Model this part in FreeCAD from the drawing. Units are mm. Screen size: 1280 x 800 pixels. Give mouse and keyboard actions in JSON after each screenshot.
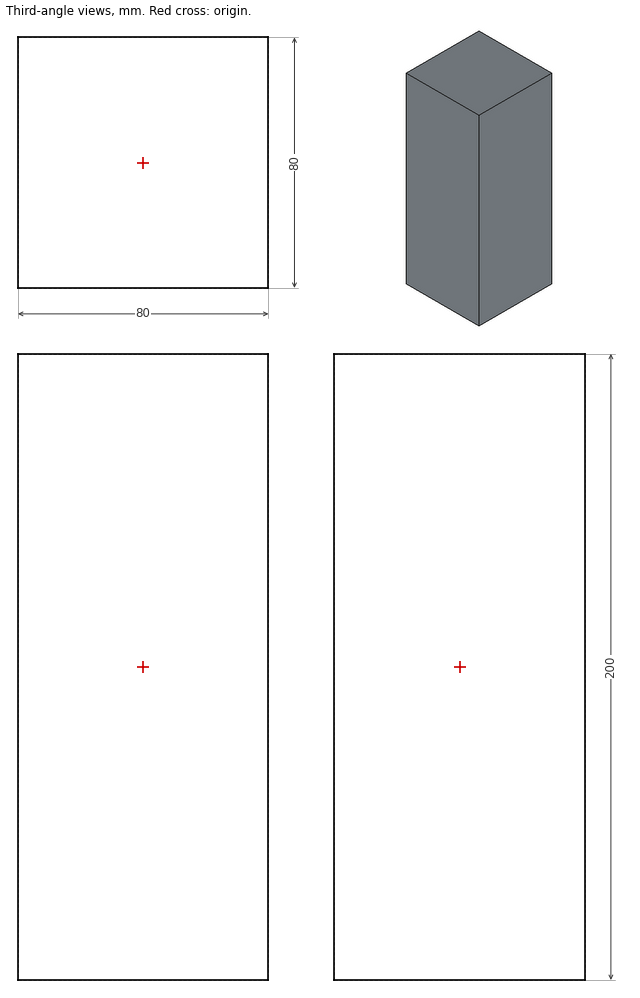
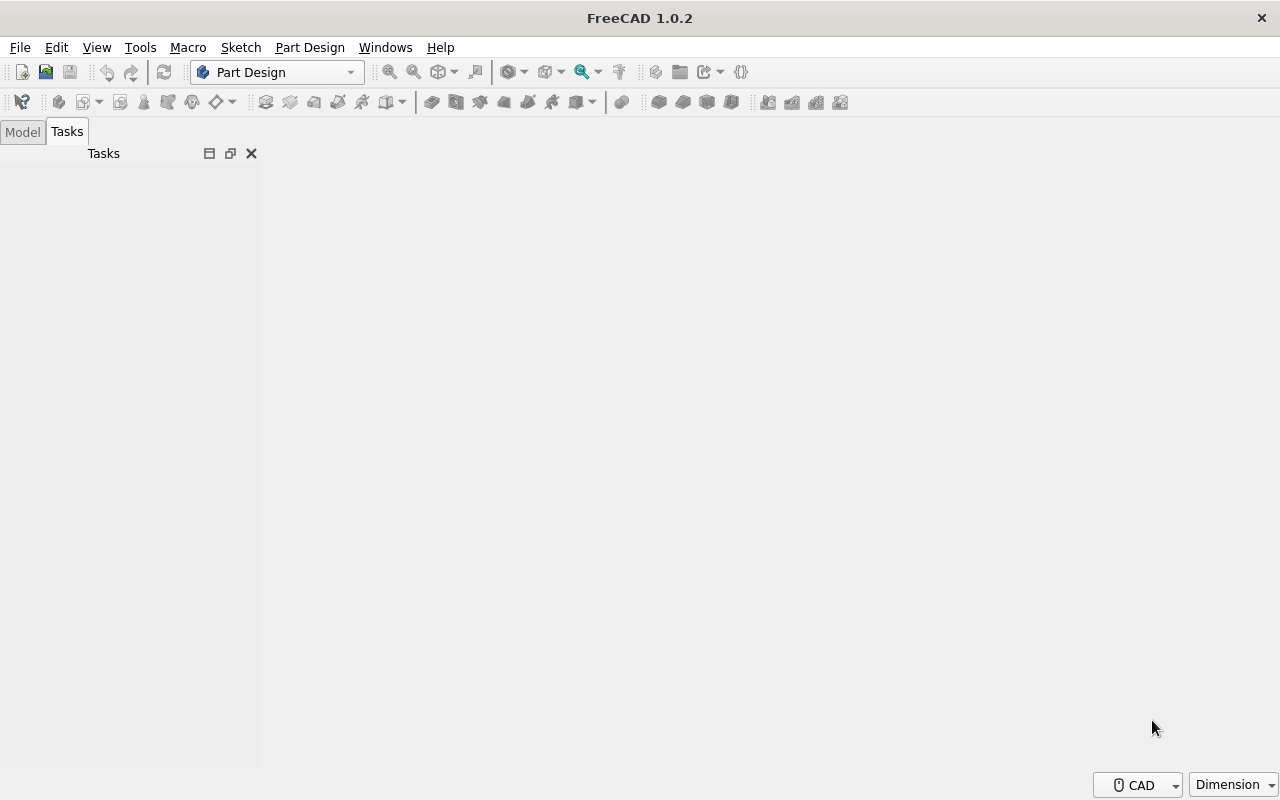
{"action": "left_click", "coordinate": [22, 72]}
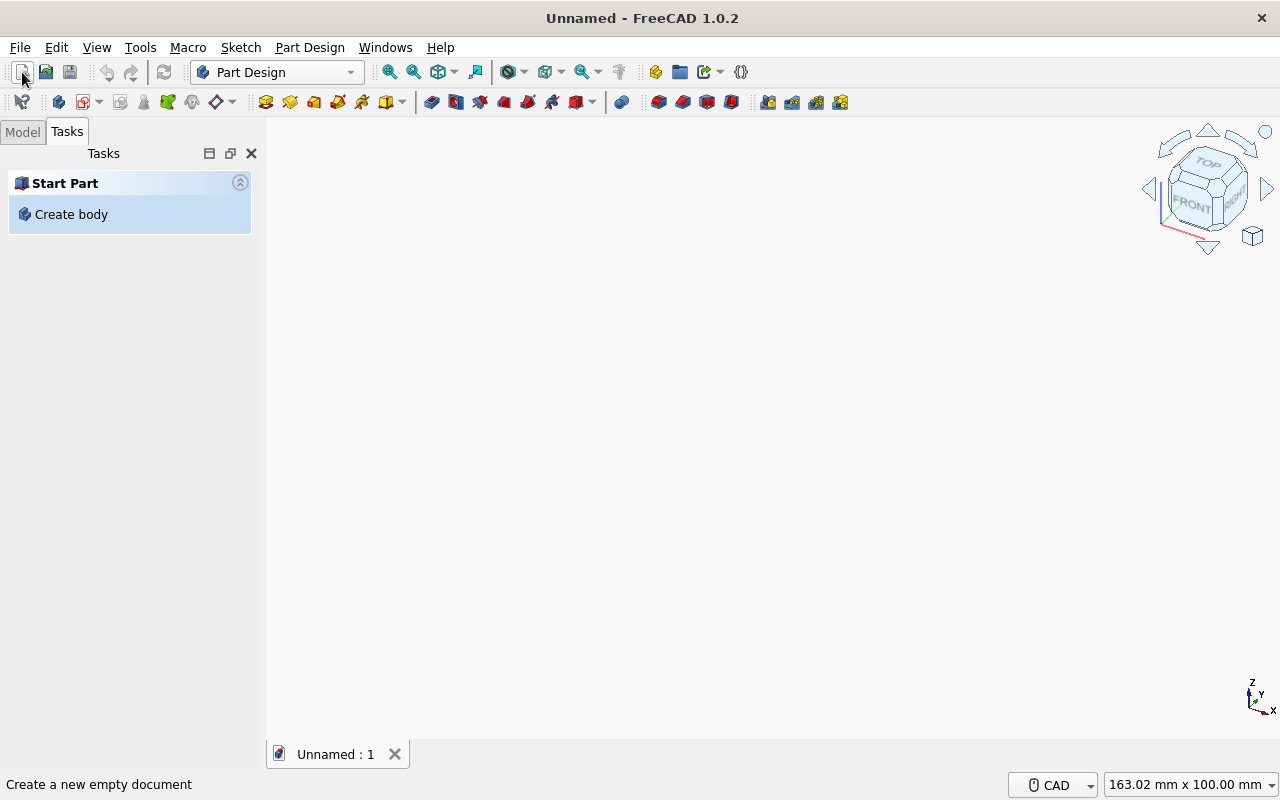
{"action": "left_click", "coordinate": [84, 102]}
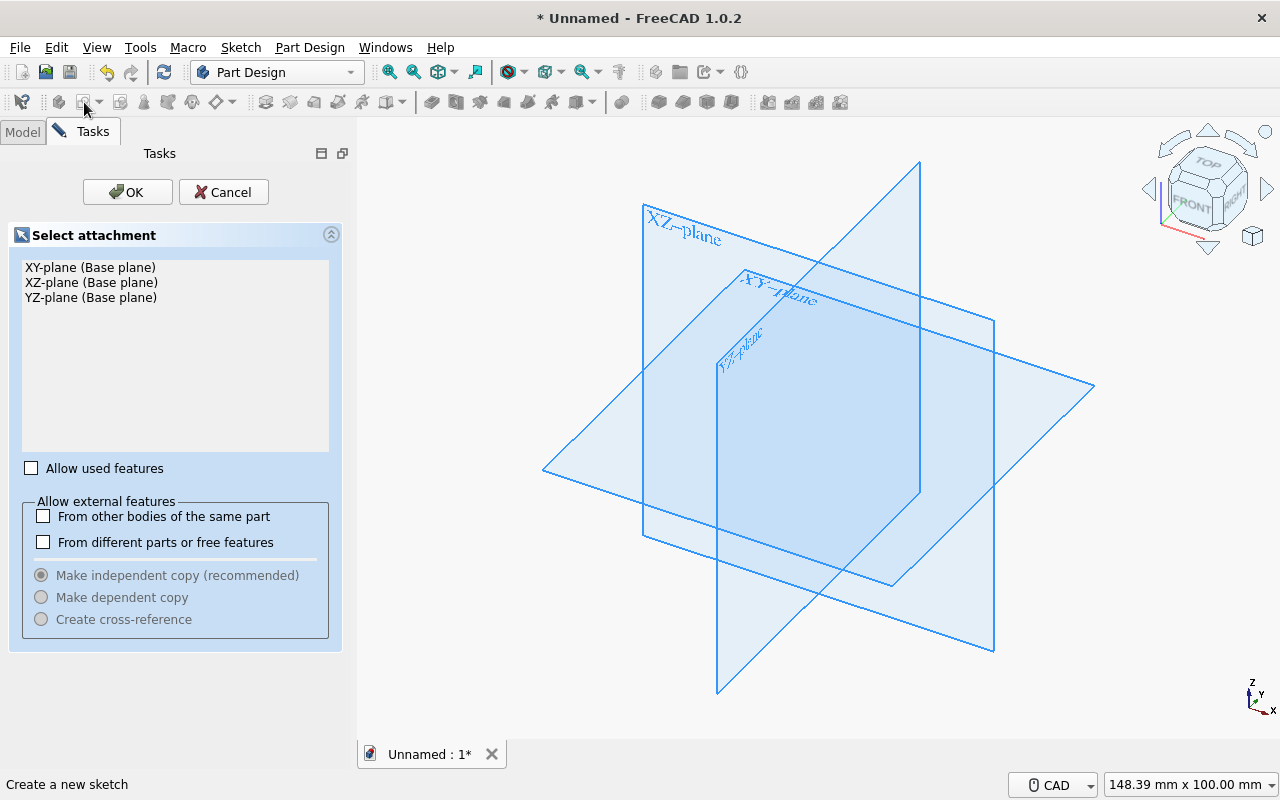
{"action": "left_click", "coordinate": [82, 268]}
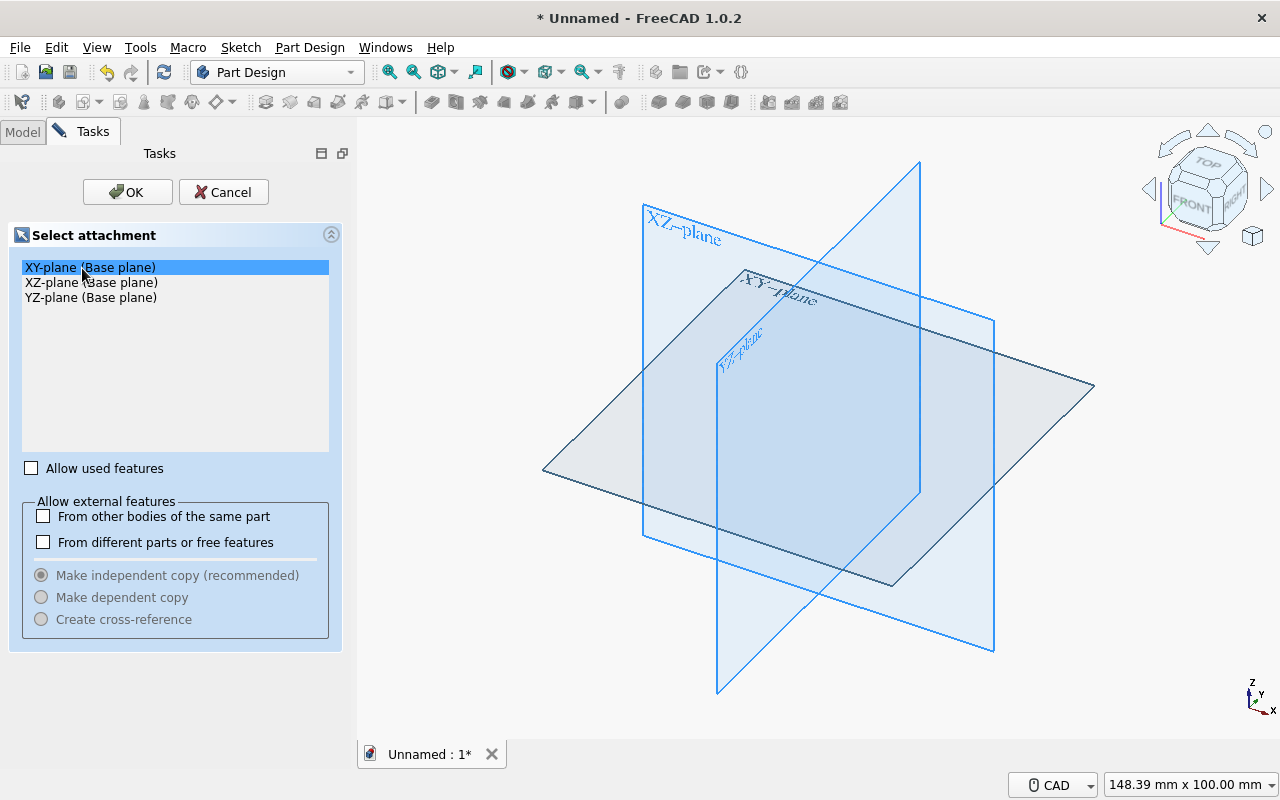
{"action": "left_click", "coordinate": [128, 192]}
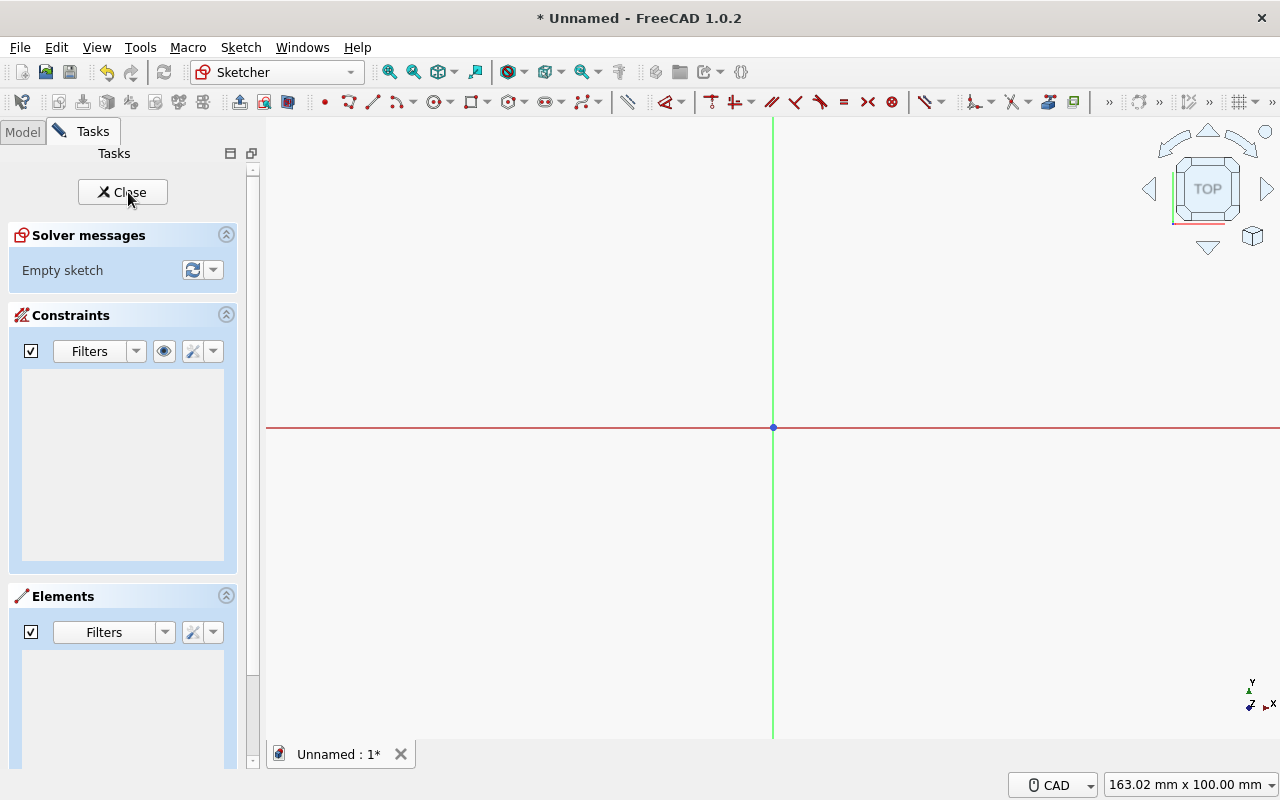
{"action": "key", "text": "g v"}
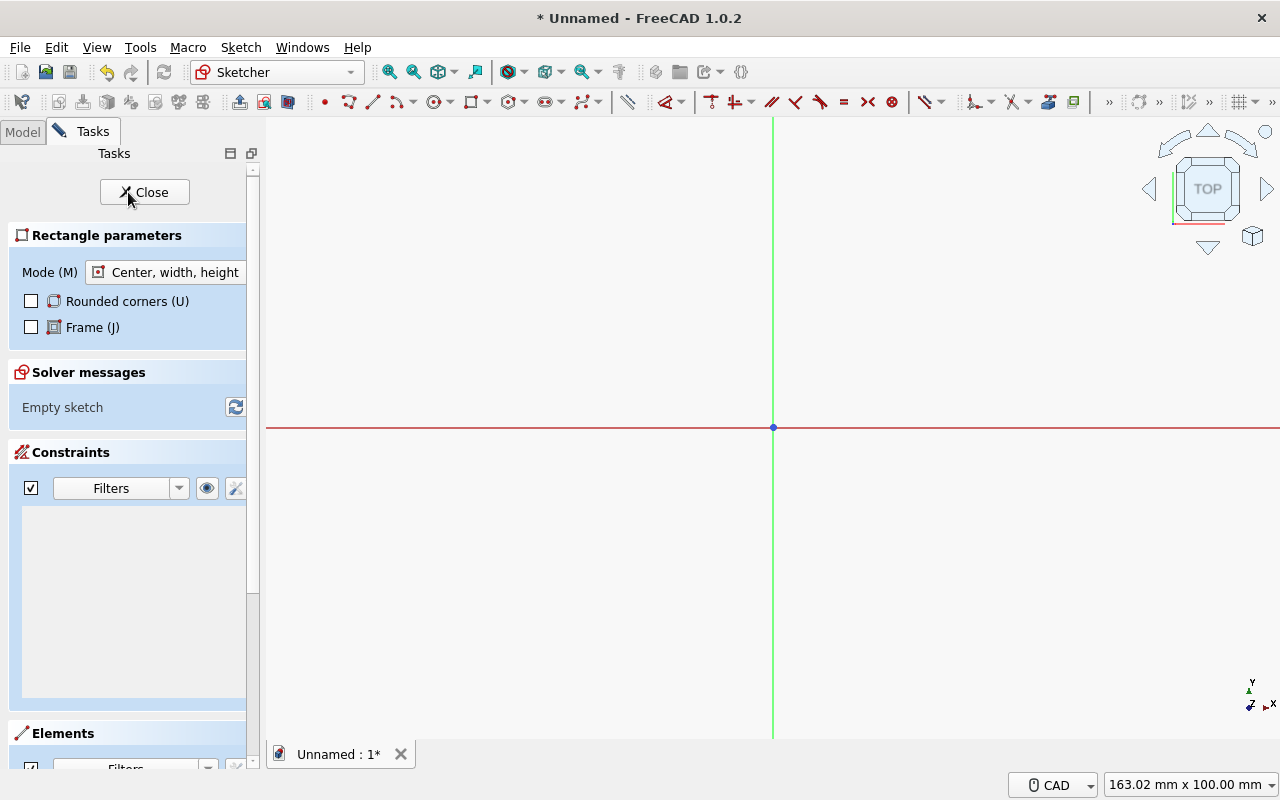
{"action": "left_click", "coordinate": [773, 428]}
{"action": "mouse_move", "coordinate": [1022, 179]}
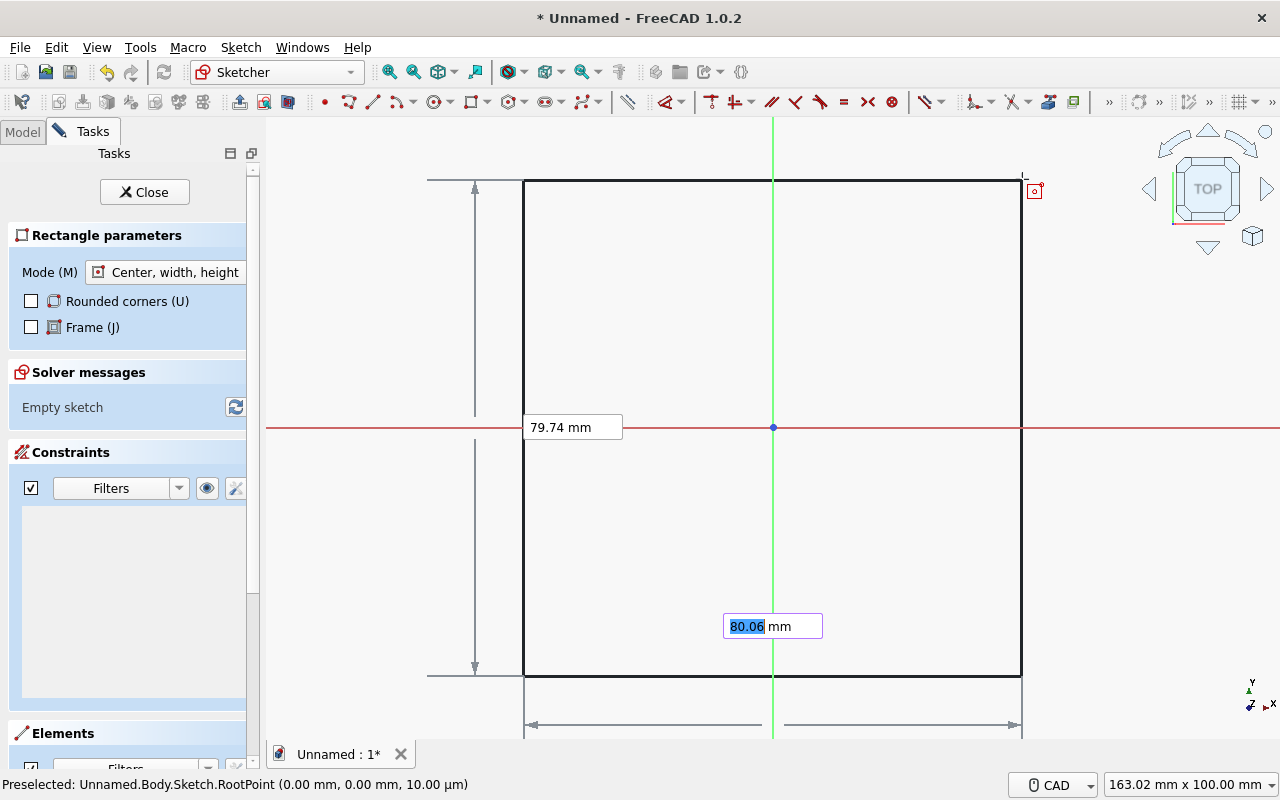
{"action": "type", "text": "80"}
{"action": "key", "text": "Tab"}
{"action": "type", "text": "80"}
{"action": "key", "text": "Return"}
{"action": "key", "text": "Escape"}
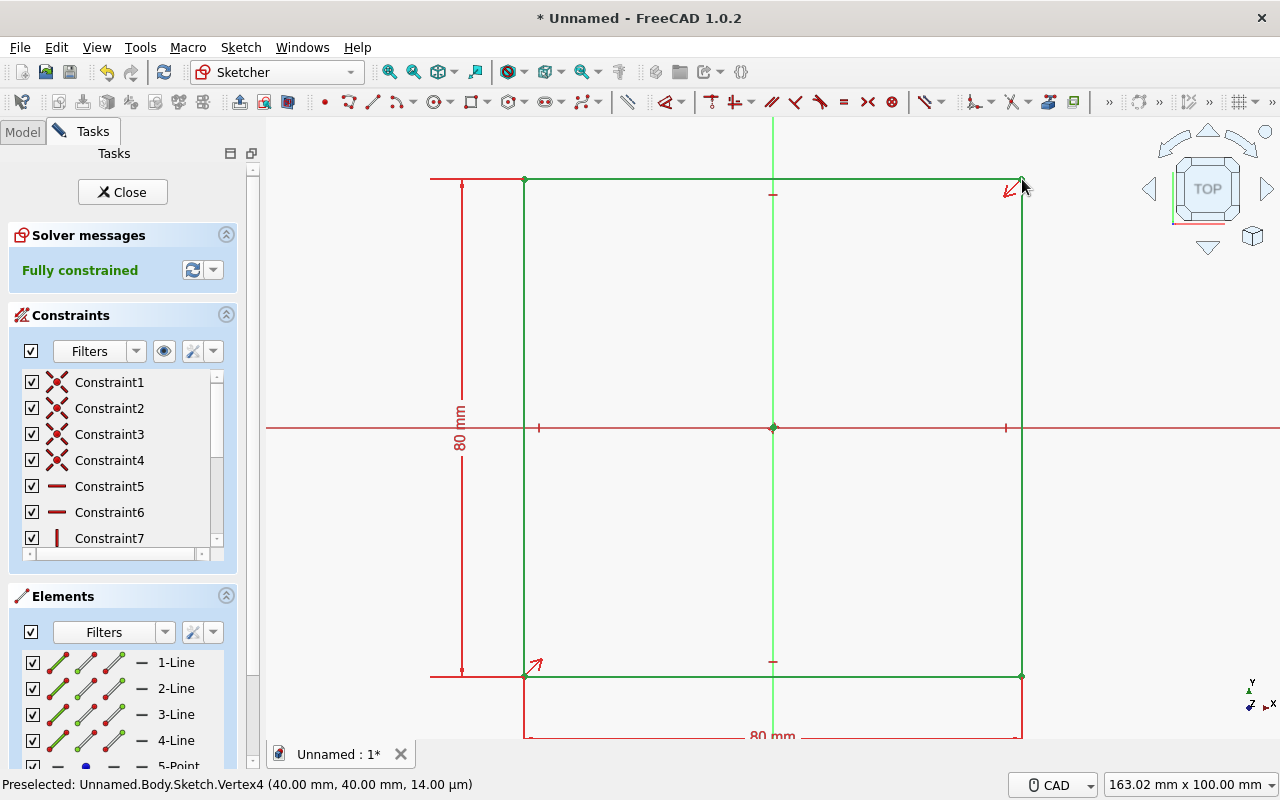
{"action": "left_click", "coordinate": [123, 192]}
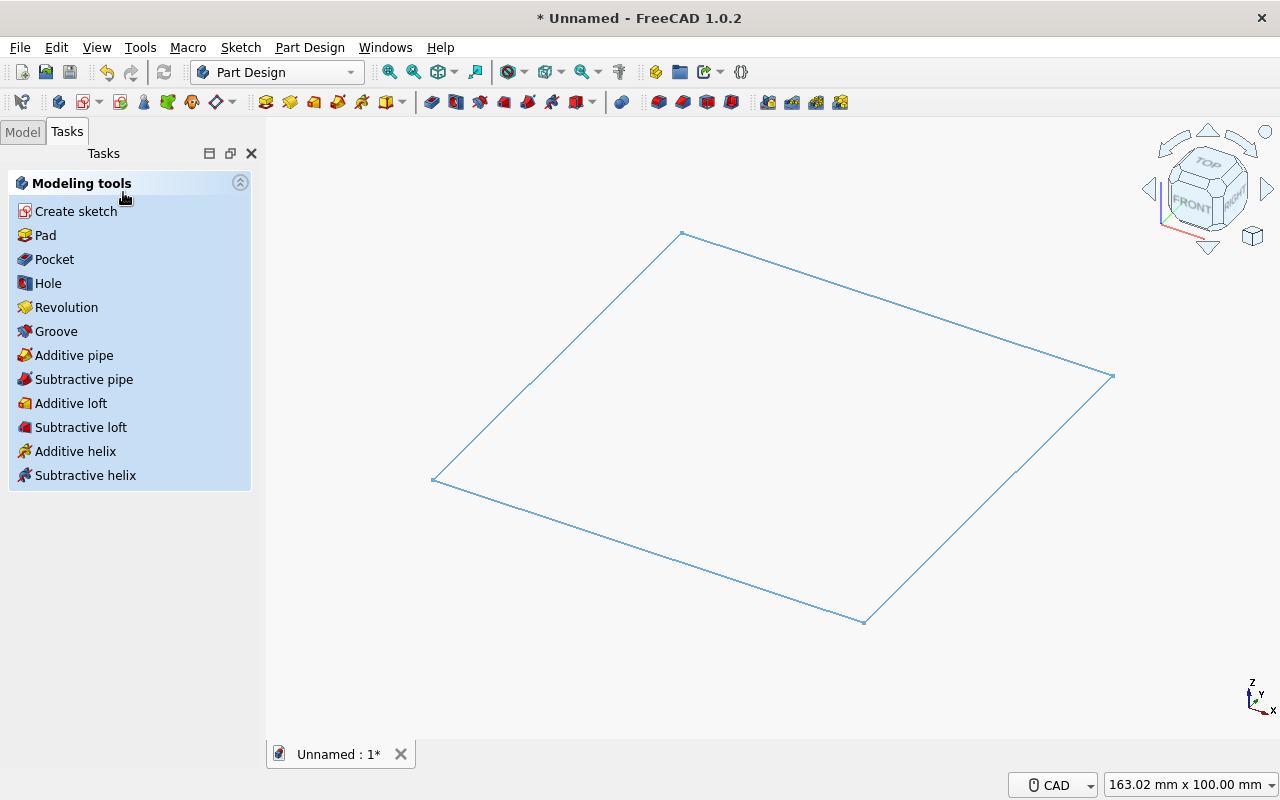
{"action": "left_click", "coordinate": [266, 102]}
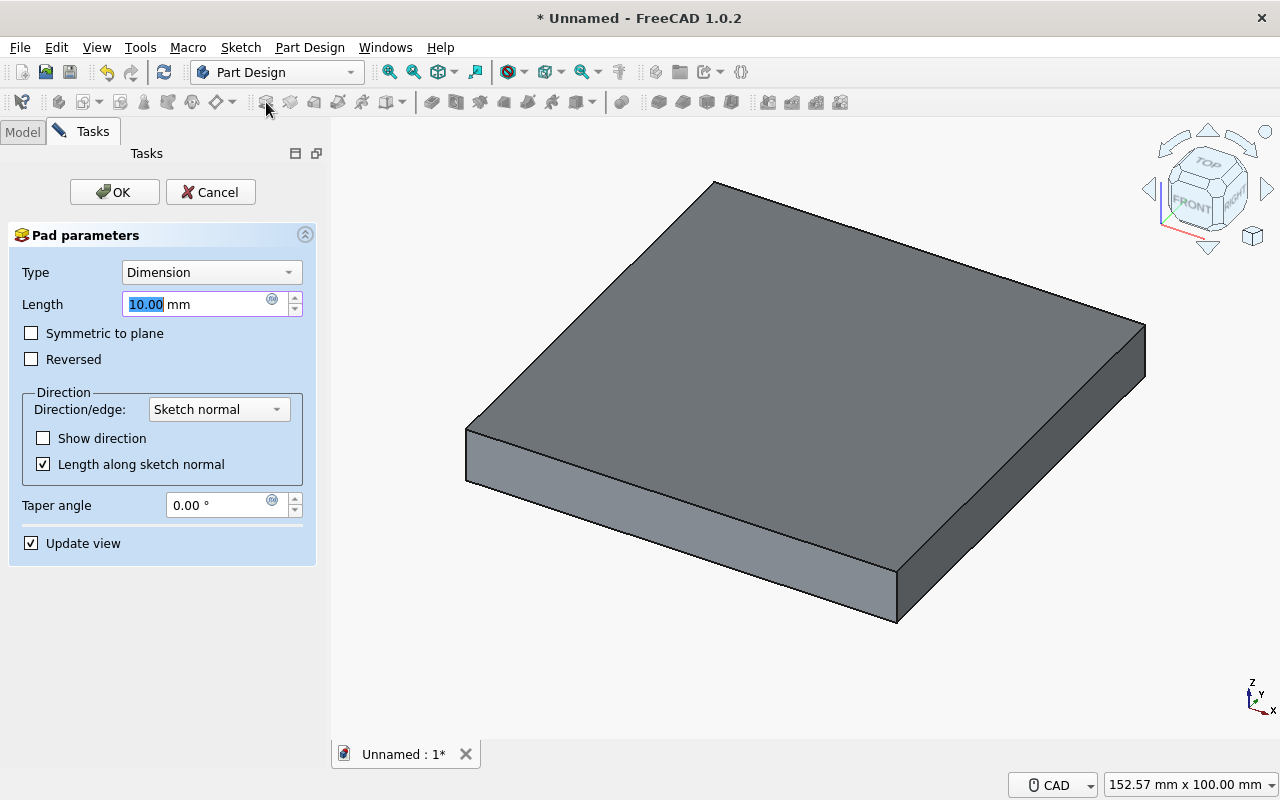
{"action": "type", "text": "200"}
{"action": "key", "text": "Tab"}